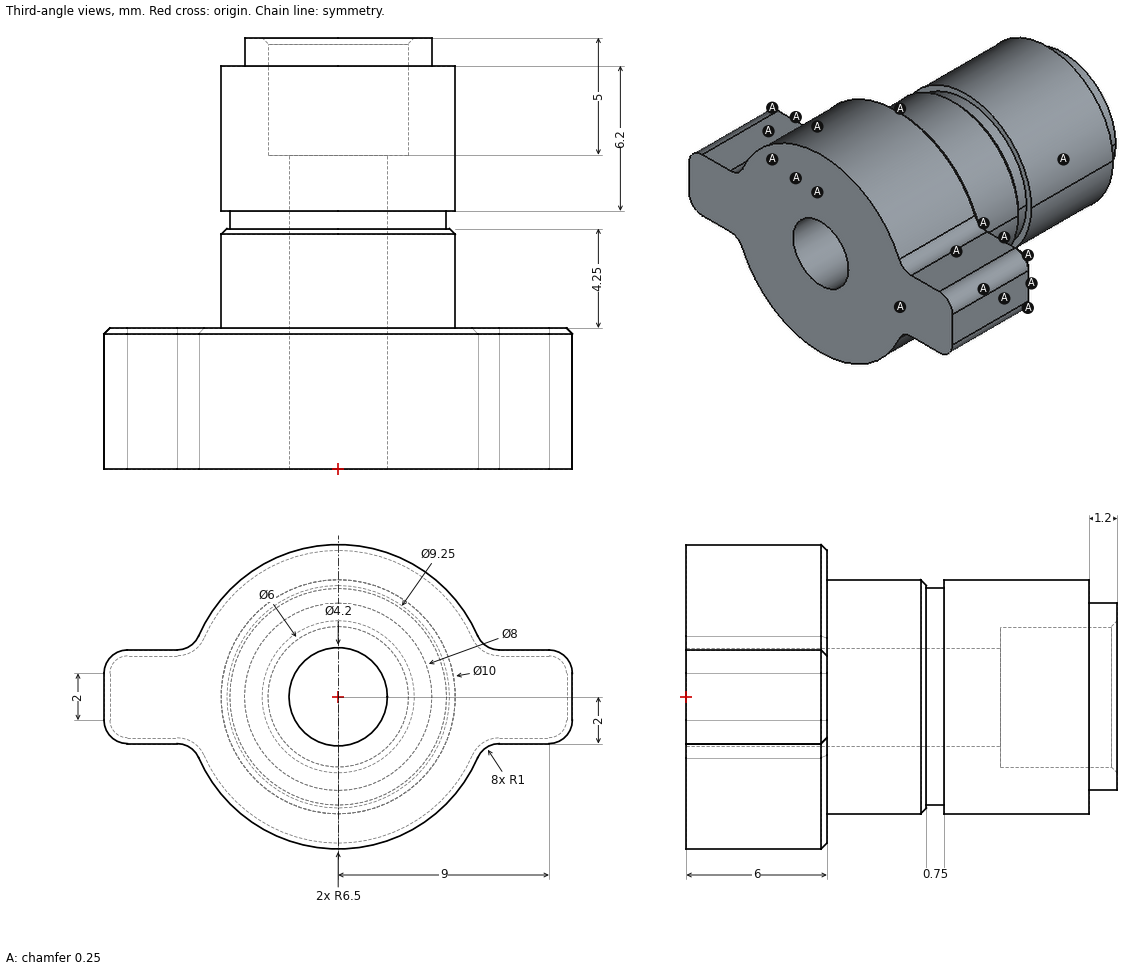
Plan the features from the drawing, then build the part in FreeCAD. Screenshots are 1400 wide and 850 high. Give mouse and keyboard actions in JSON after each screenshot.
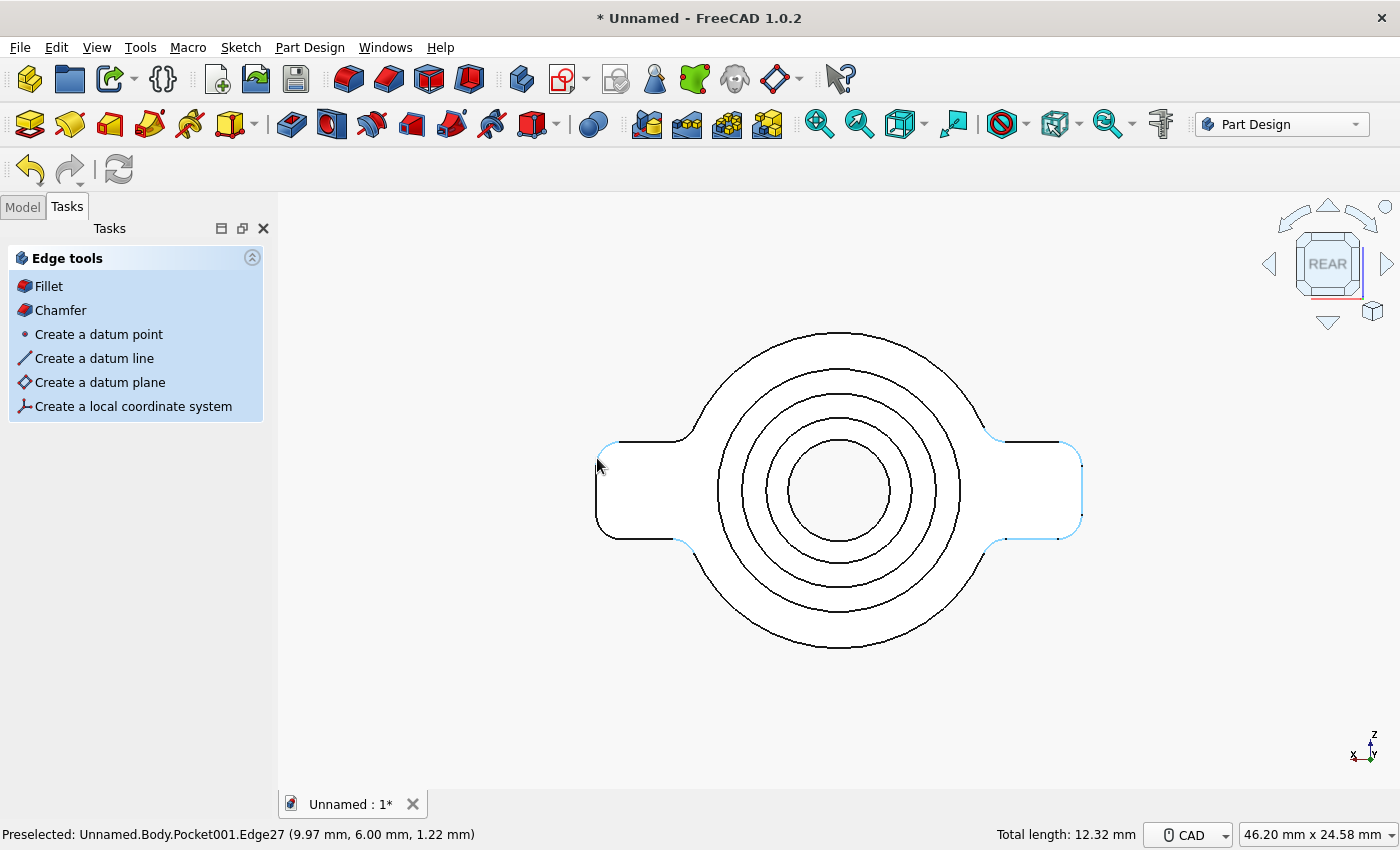
{"action": "left_click", "coordinate": [603, 531], "text": "ctrl"}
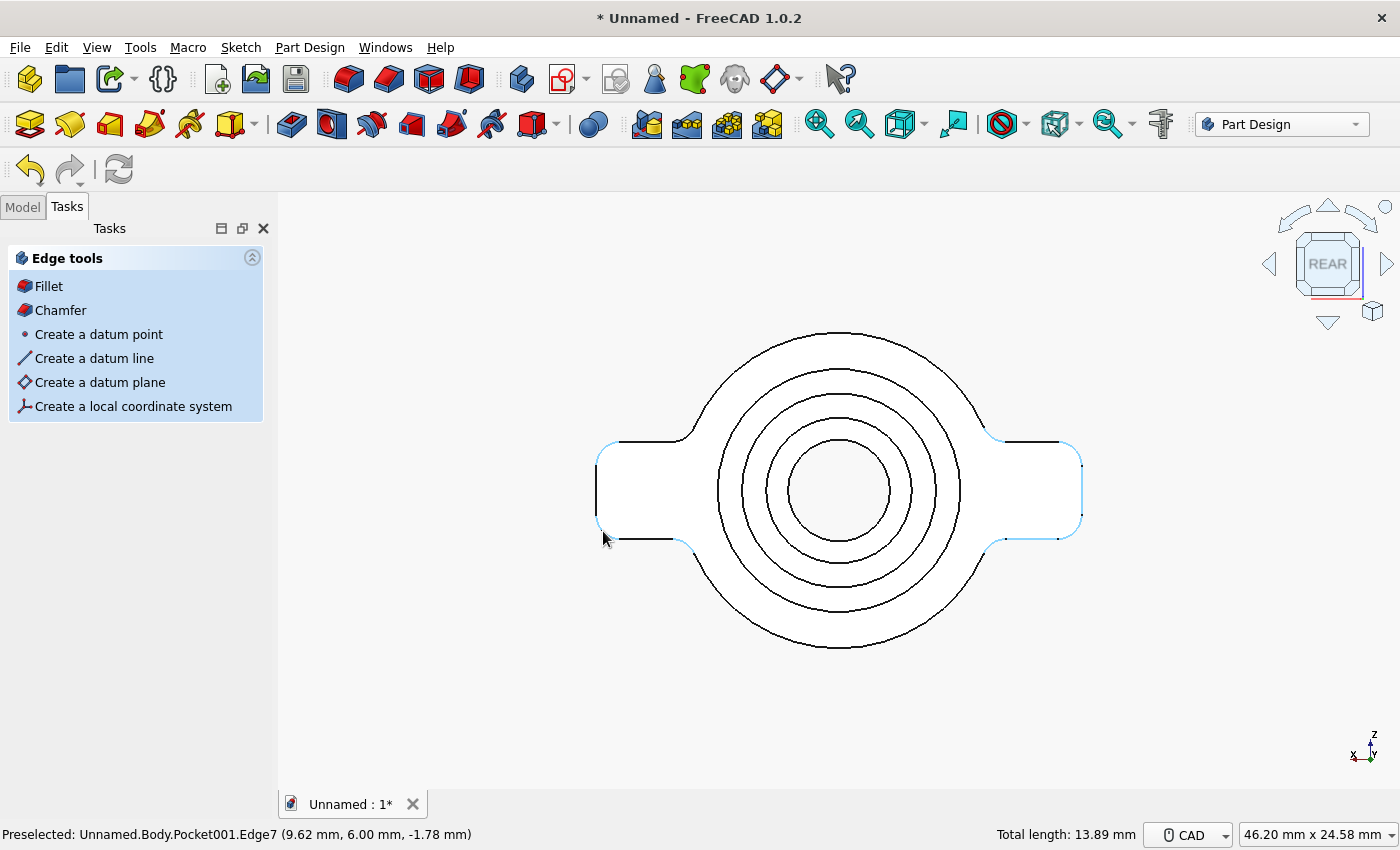
{"action": "left_click", "coordinate": [646, 538], "text": "ctrl"}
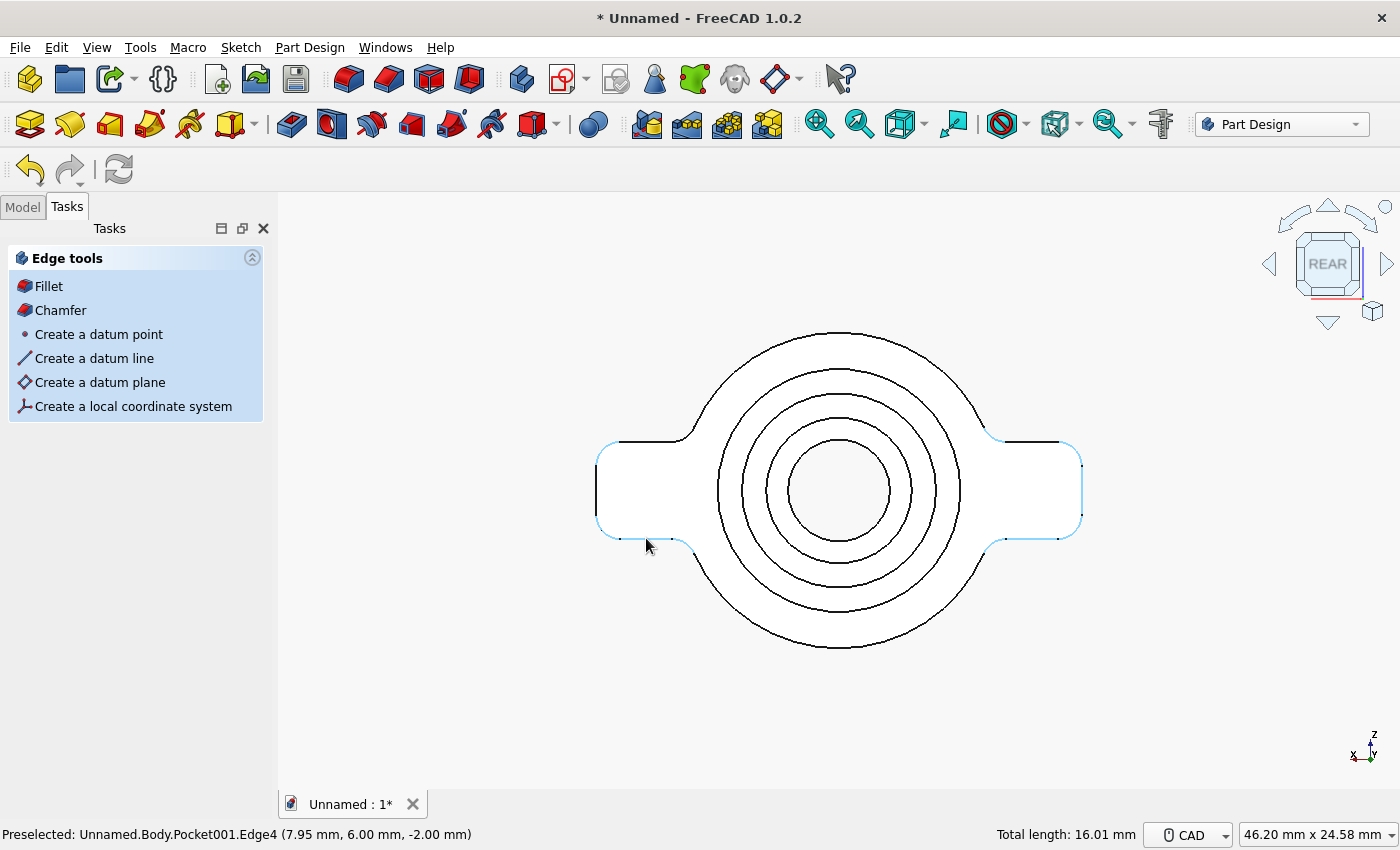
{"action": "left_click", "coordinate": [898, 447], "text": "ctrl"}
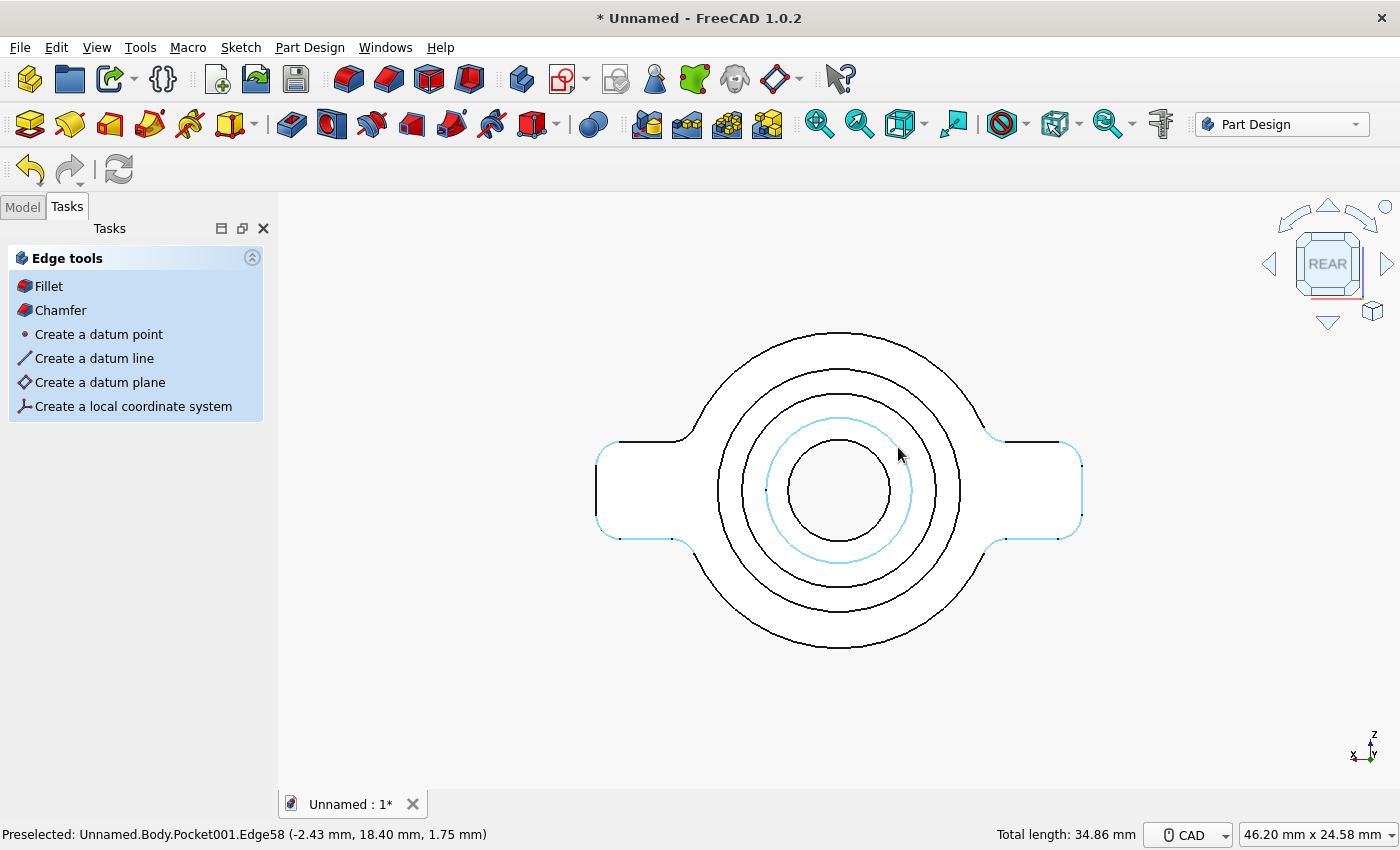
{"action": "left_click", "coordinate": [839, 647], "text": "ctrl"}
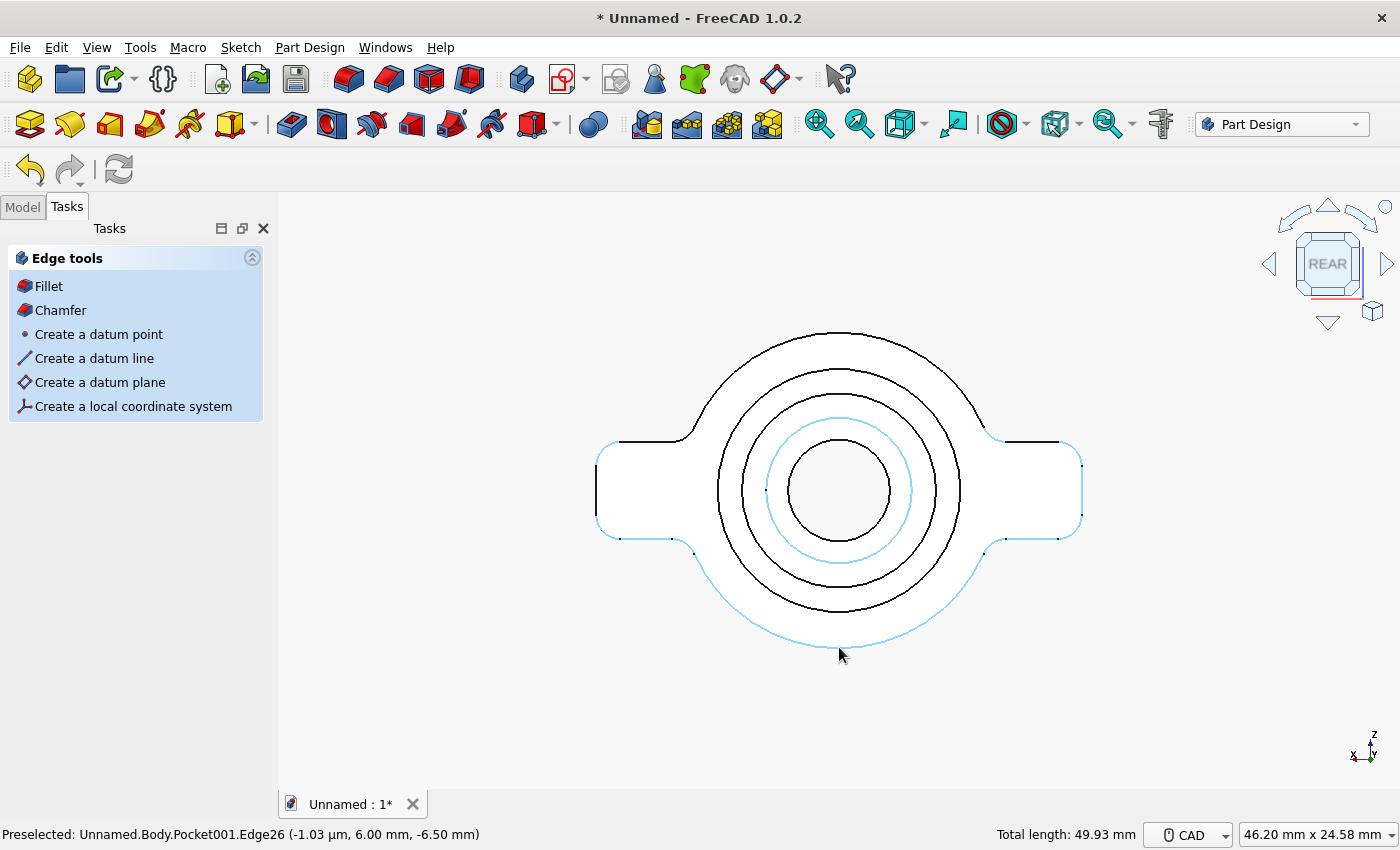
{"action": "key", "text": "0"}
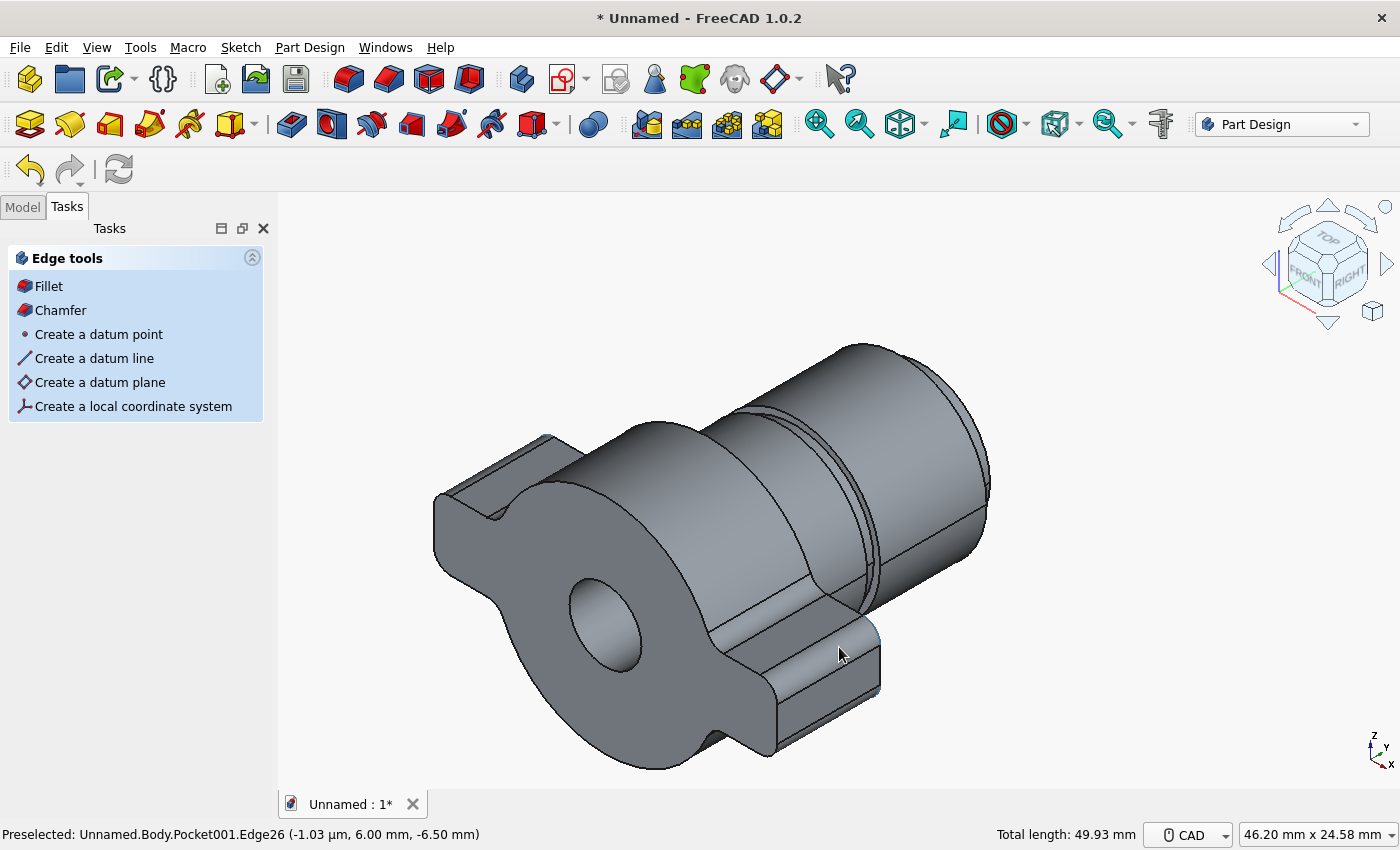
{"action": "left_click", "coordinate": [820, 124]}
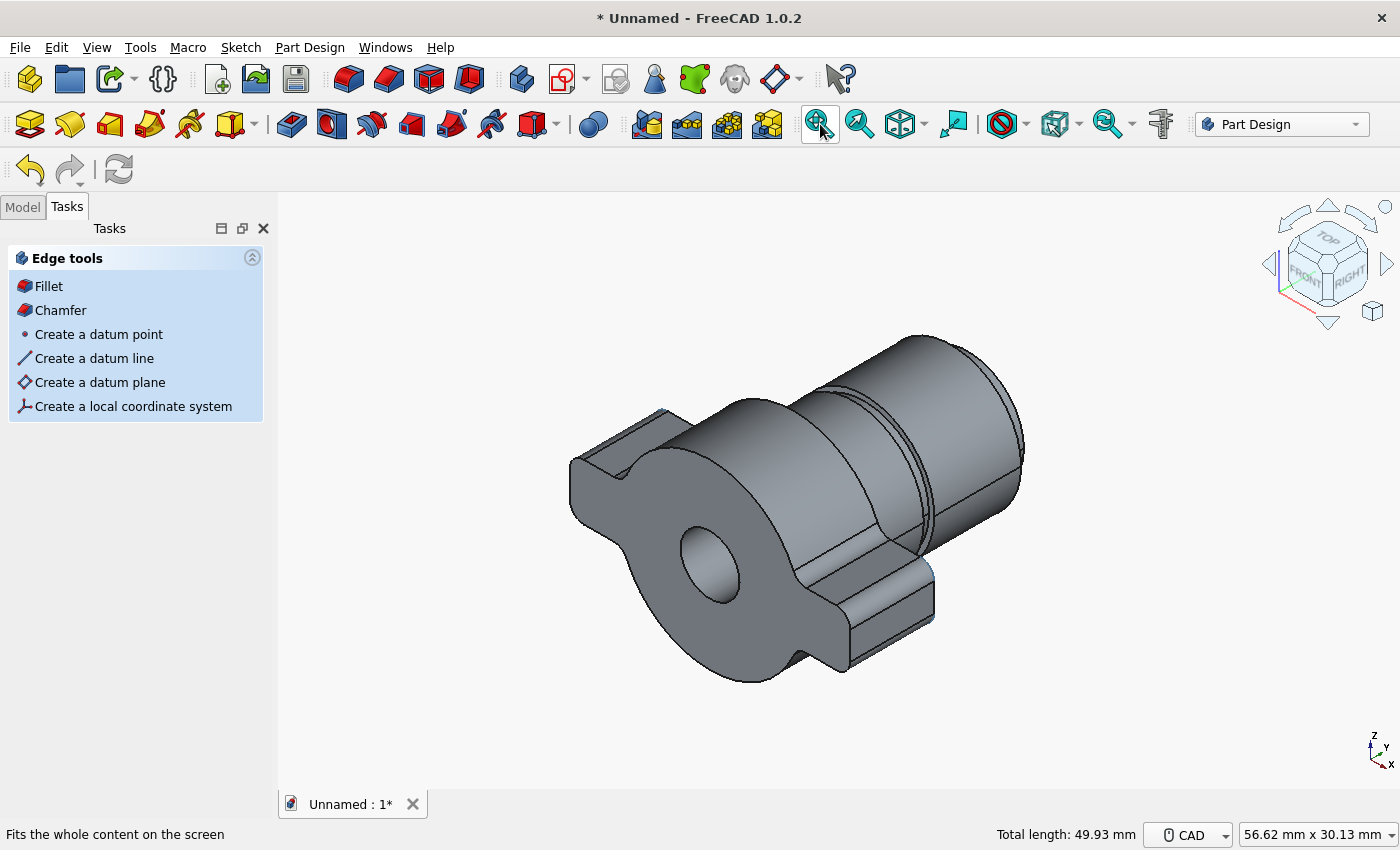
{"action": "key", "text": "2"}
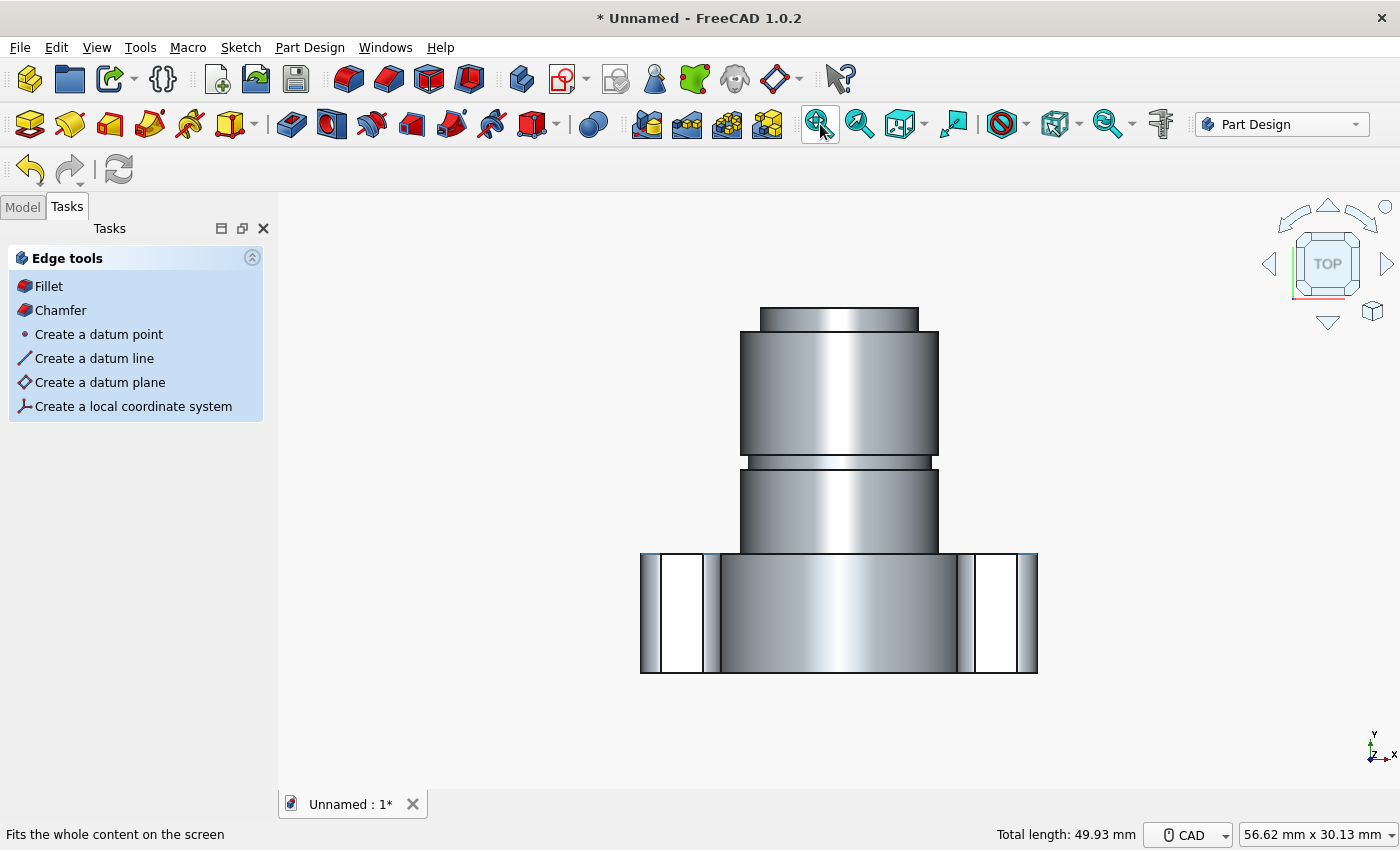
{"action": "left_click", "coordinate": [682, 553], "text": "ctrl"}